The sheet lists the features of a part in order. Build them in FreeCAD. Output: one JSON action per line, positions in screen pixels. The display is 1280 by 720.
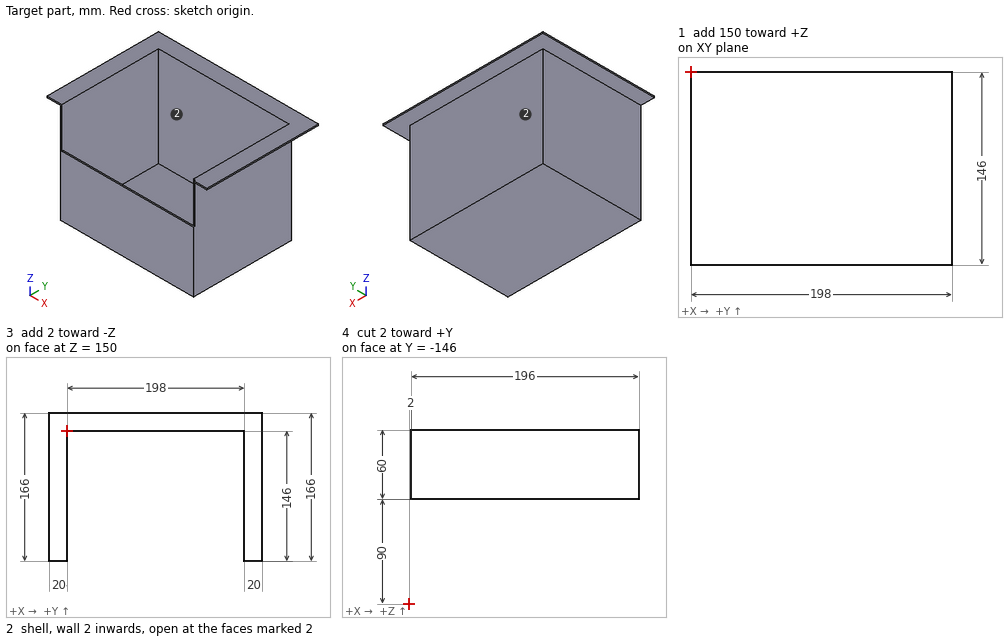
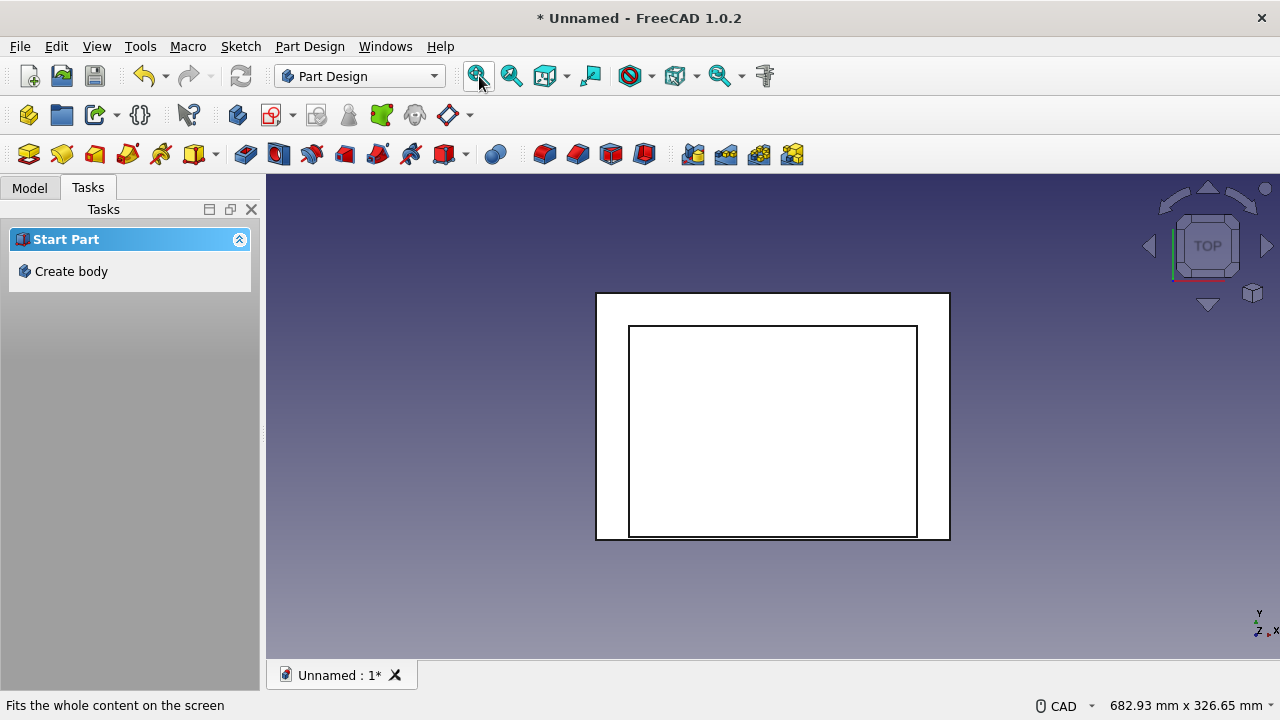
{"action": "key", "text": "0"}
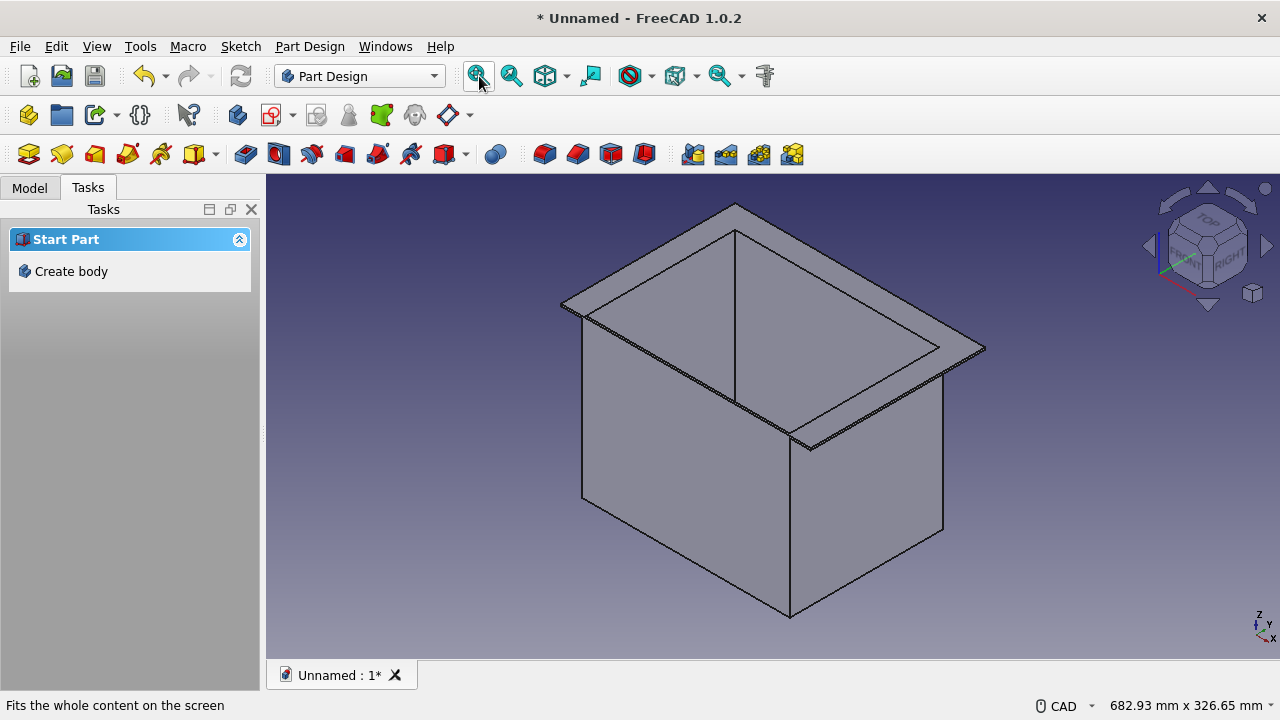
{"action": "left_click", "coordinate": [686, 466]}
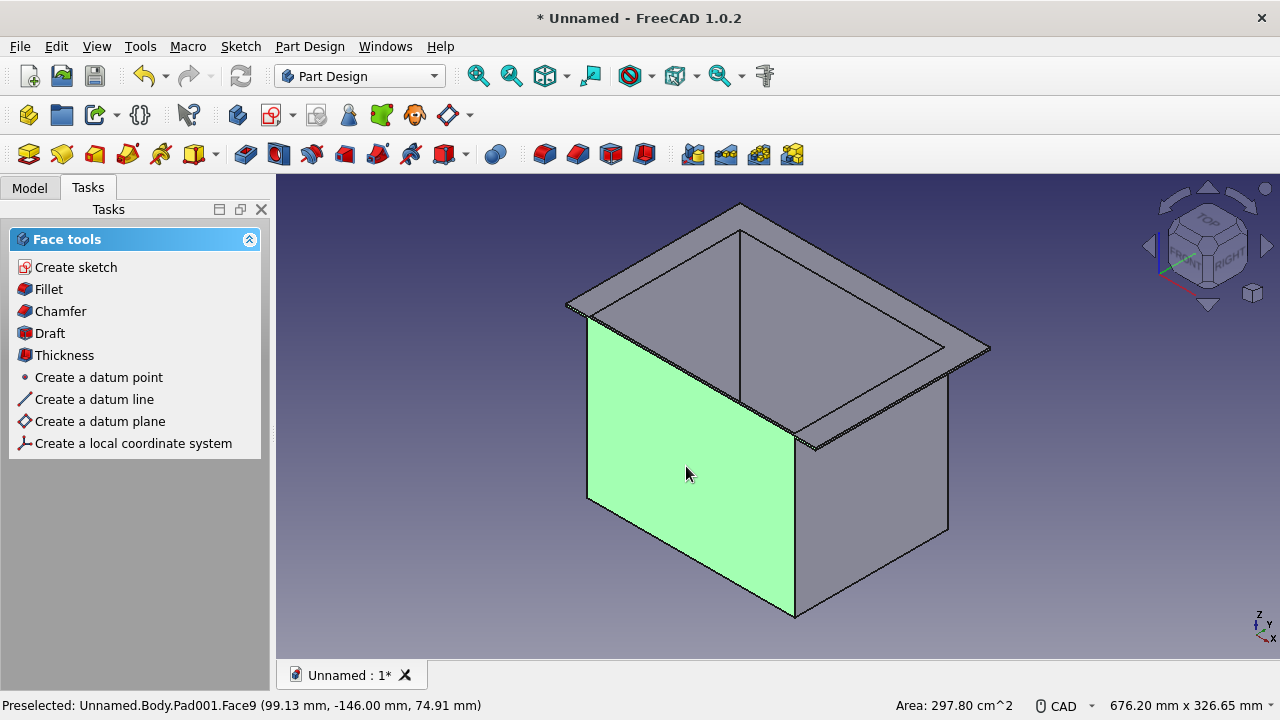
{"action": "left_click", "coordinate": [270, 116]}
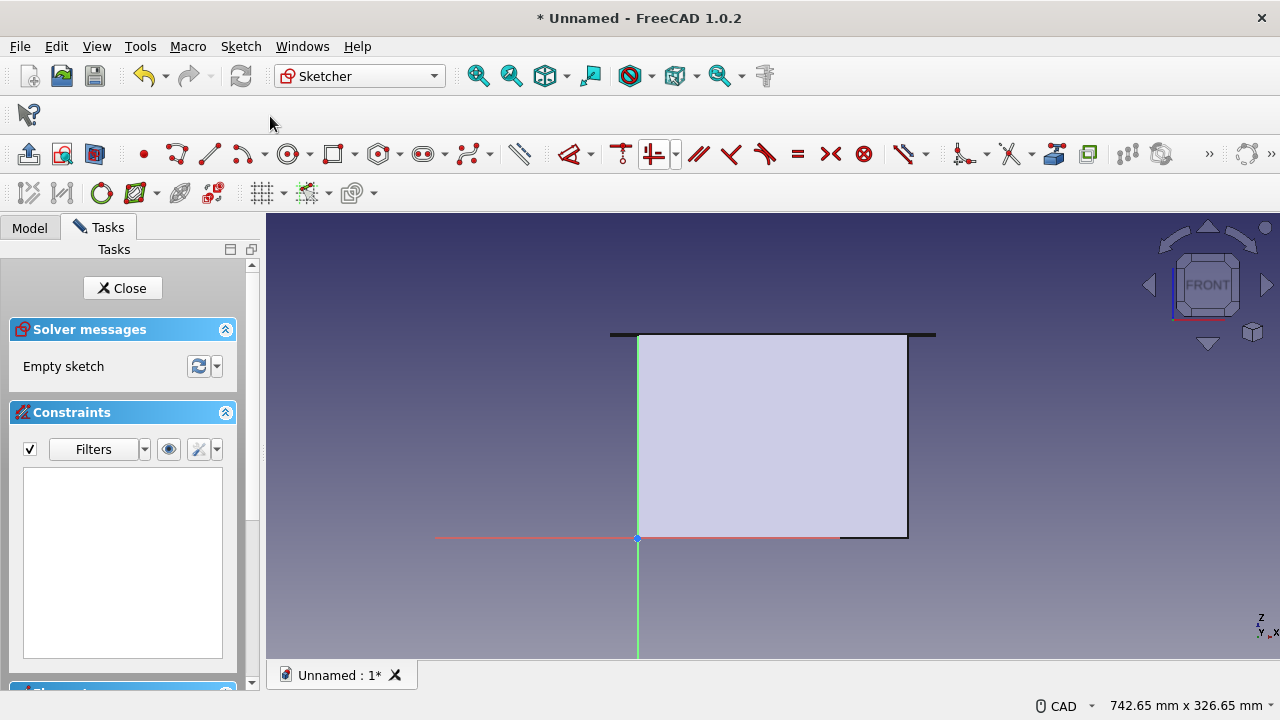
{"action": "left_click", "coordinate": [332, 154]}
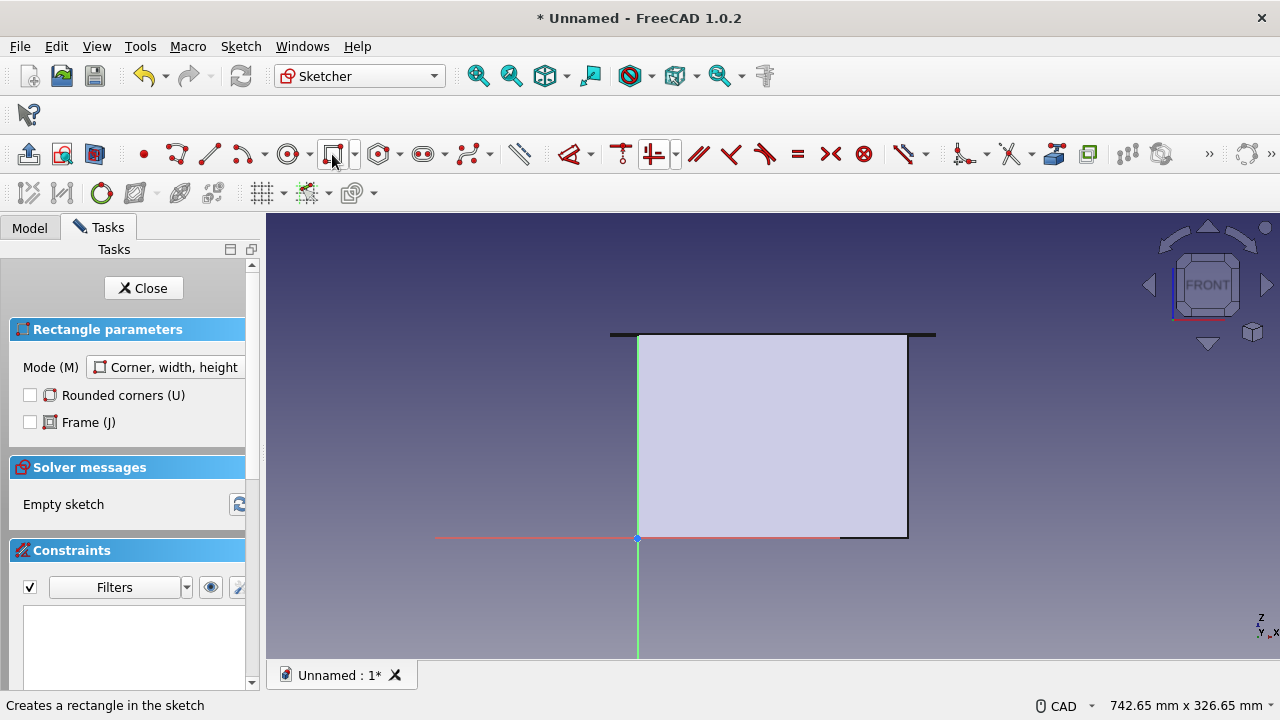
{"action": "scroll", "coordinate": [641, 334], "scroll_direction": "up", "scroll_amount": 9}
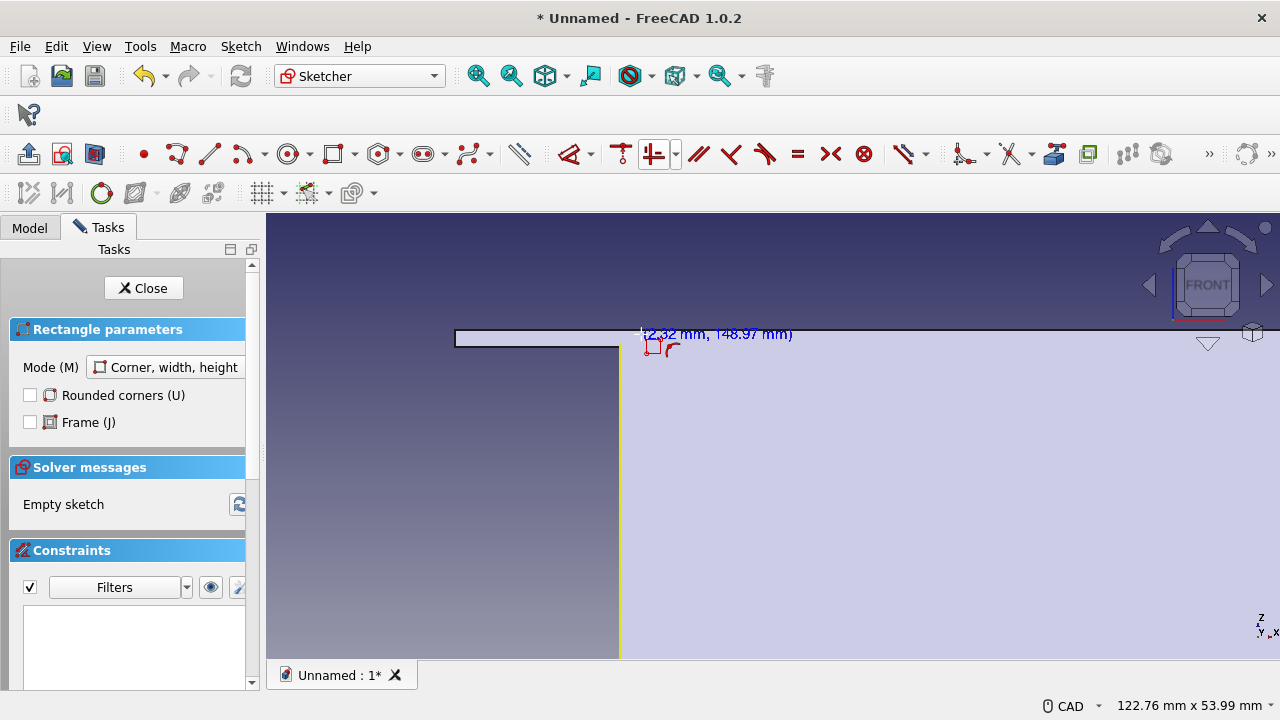
{"action": "left_click", "coordinate": [636, 330]}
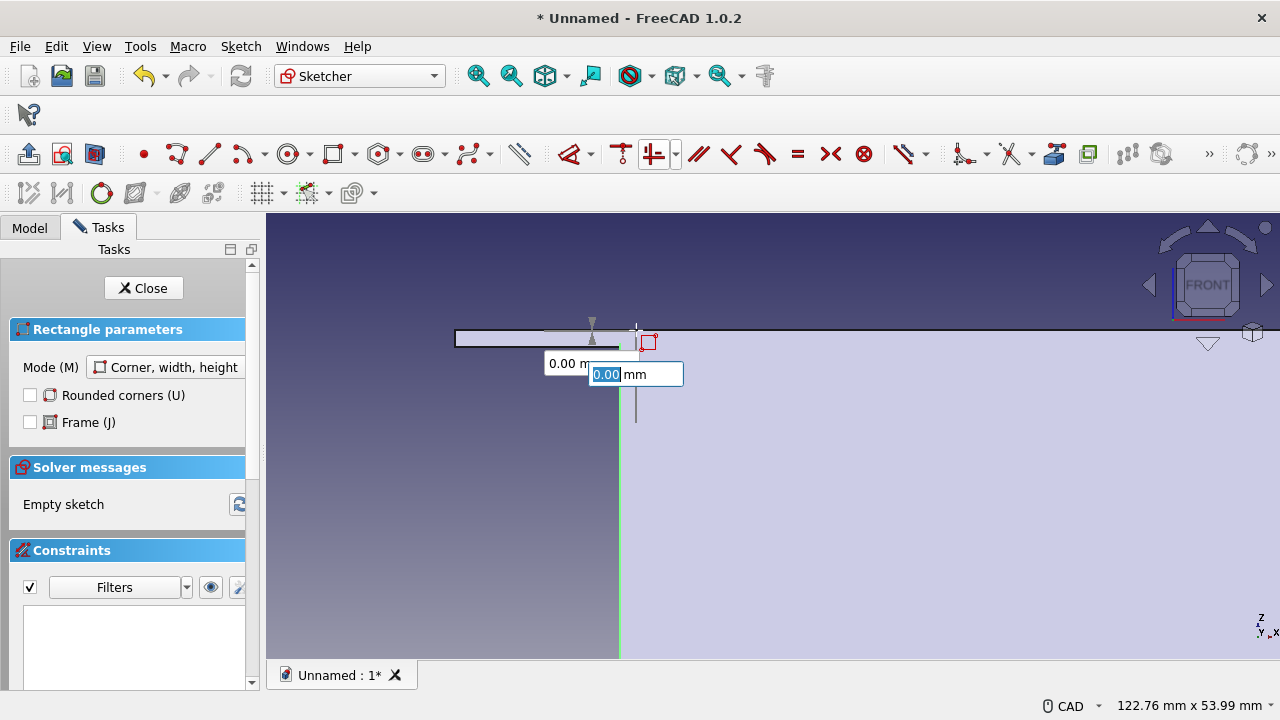
{"action": "scroll", "coordinate": [519, 306], "scroll_direction": "down", "scroll_amount": 8}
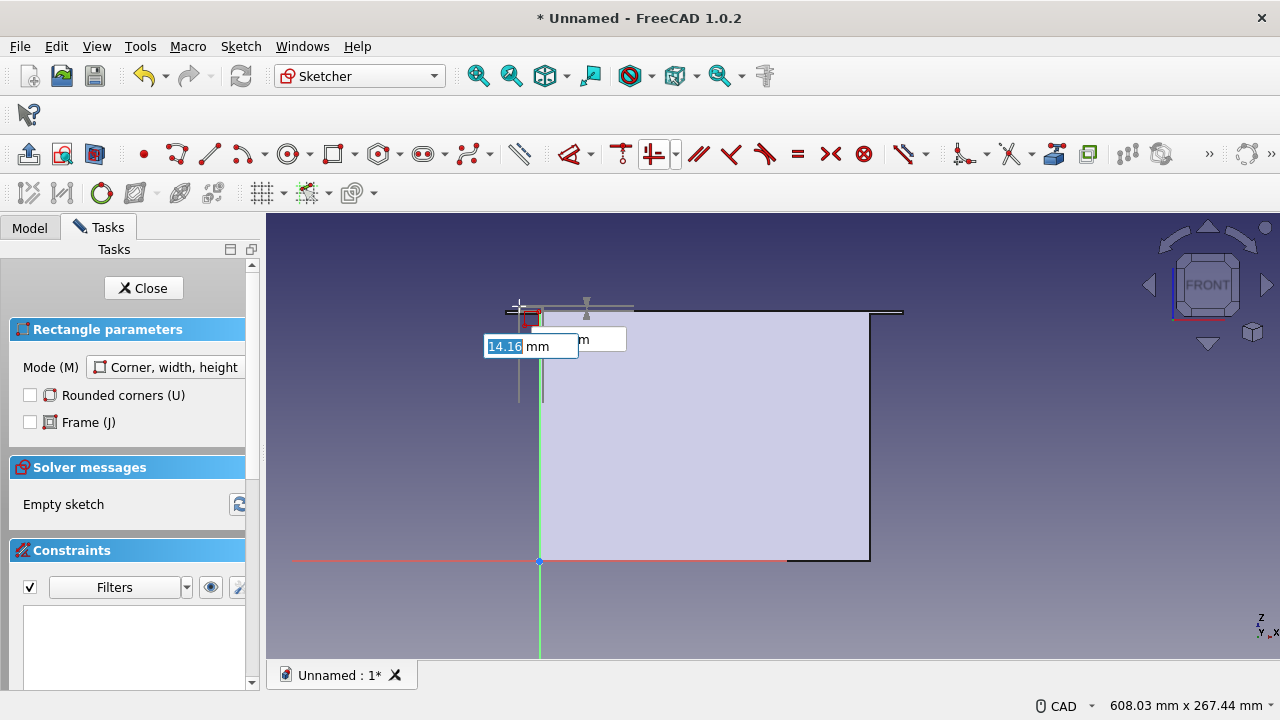
{"action": "left_click", "coordinate": [870, 411]}
{"action": "key", "text": "Escape"}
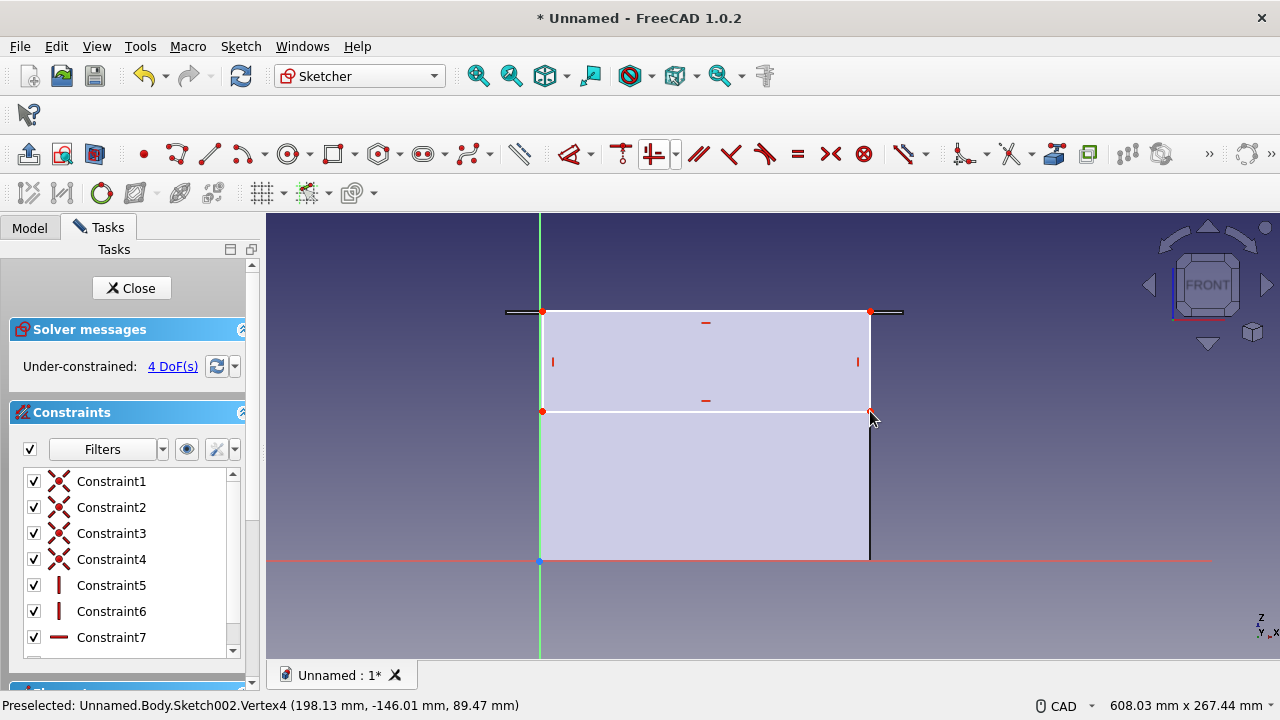
{"action": "left_click", "coordinate": [568, 154]}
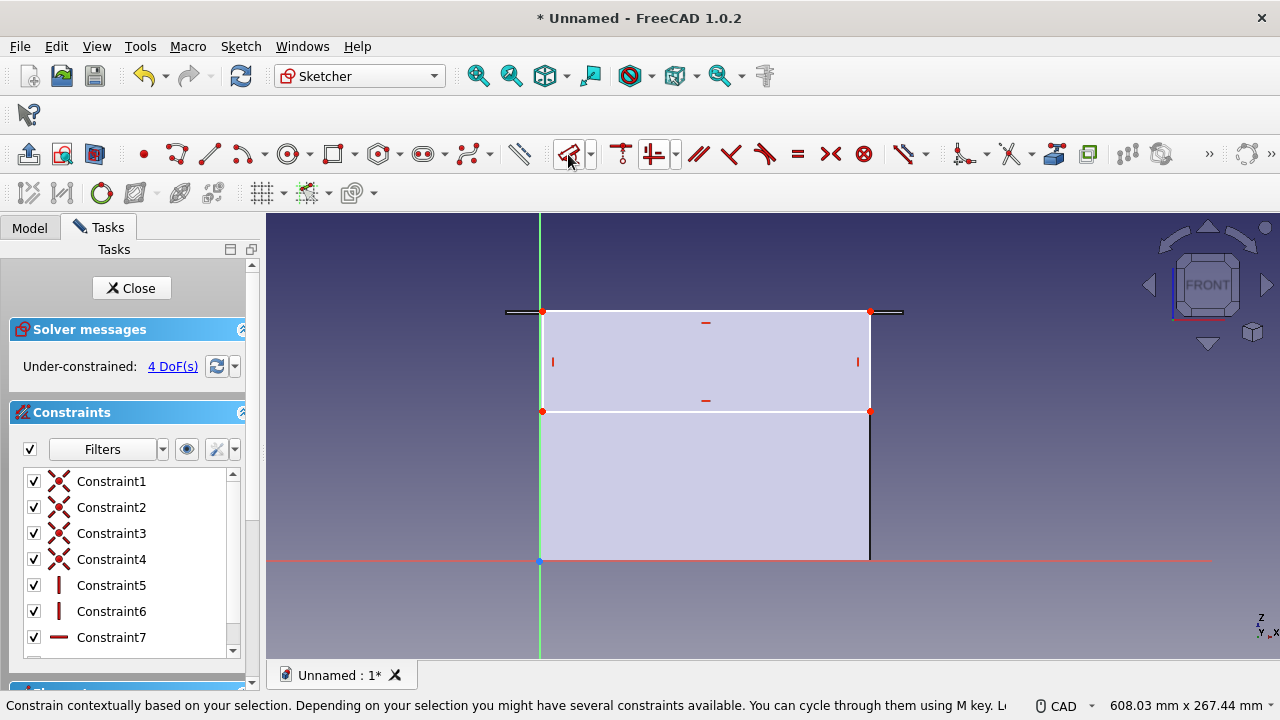
{"action": "left_click", "coordinate": [543, 341]}
{"action": "left_click", "coordinate": [509, 362]}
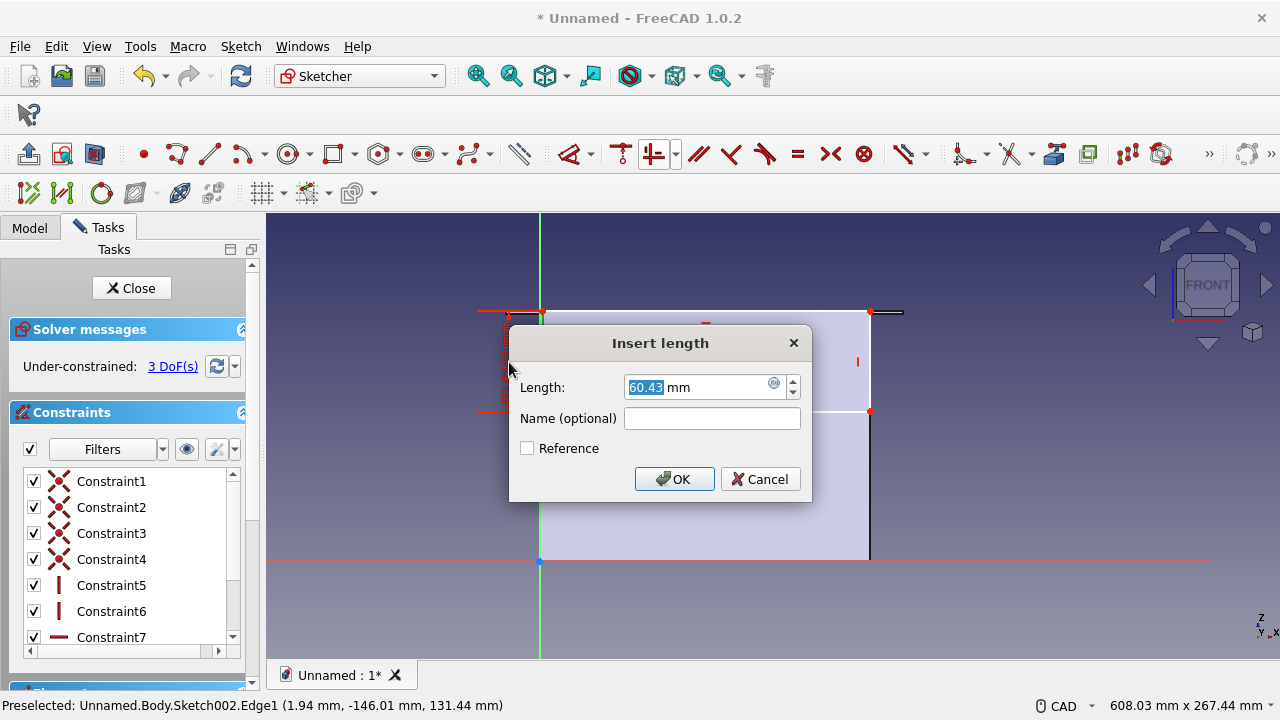
{"action": "type", "text": "60"}
{"action": "key", "text": "Return"}